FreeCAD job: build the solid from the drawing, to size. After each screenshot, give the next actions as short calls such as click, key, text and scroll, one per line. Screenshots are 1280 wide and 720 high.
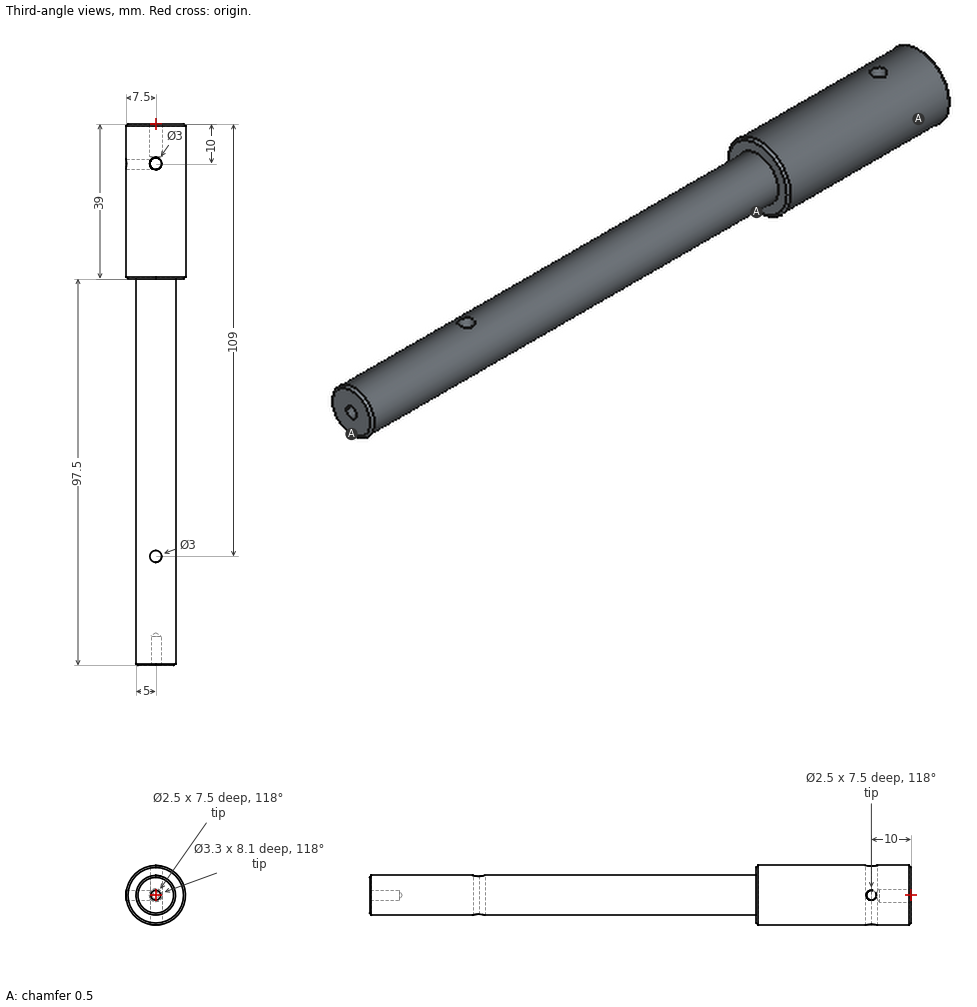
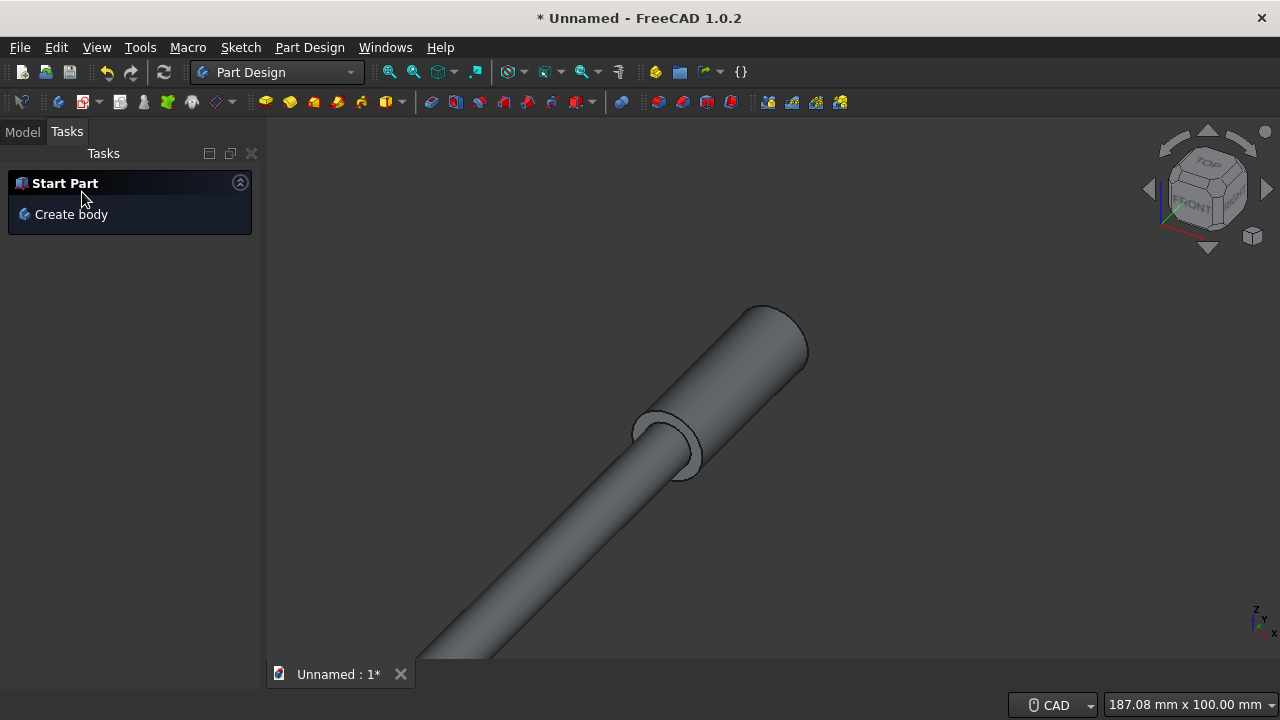
click(390, 72)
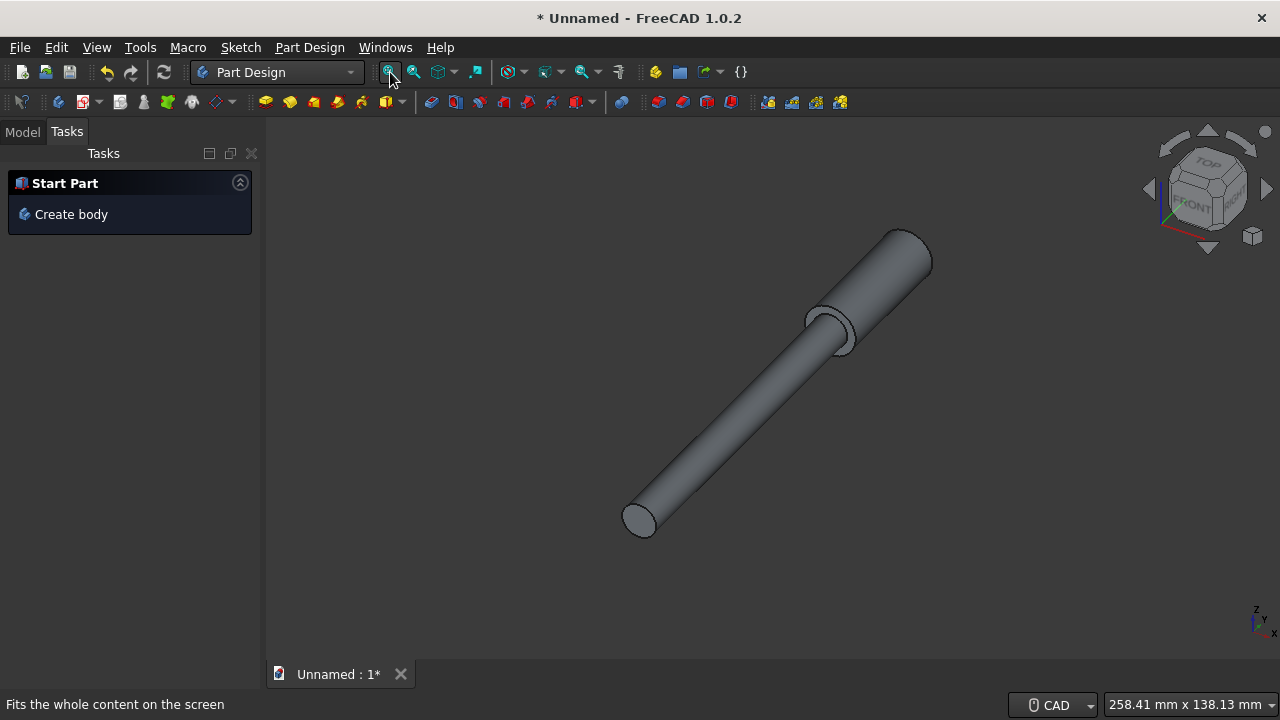
key(4)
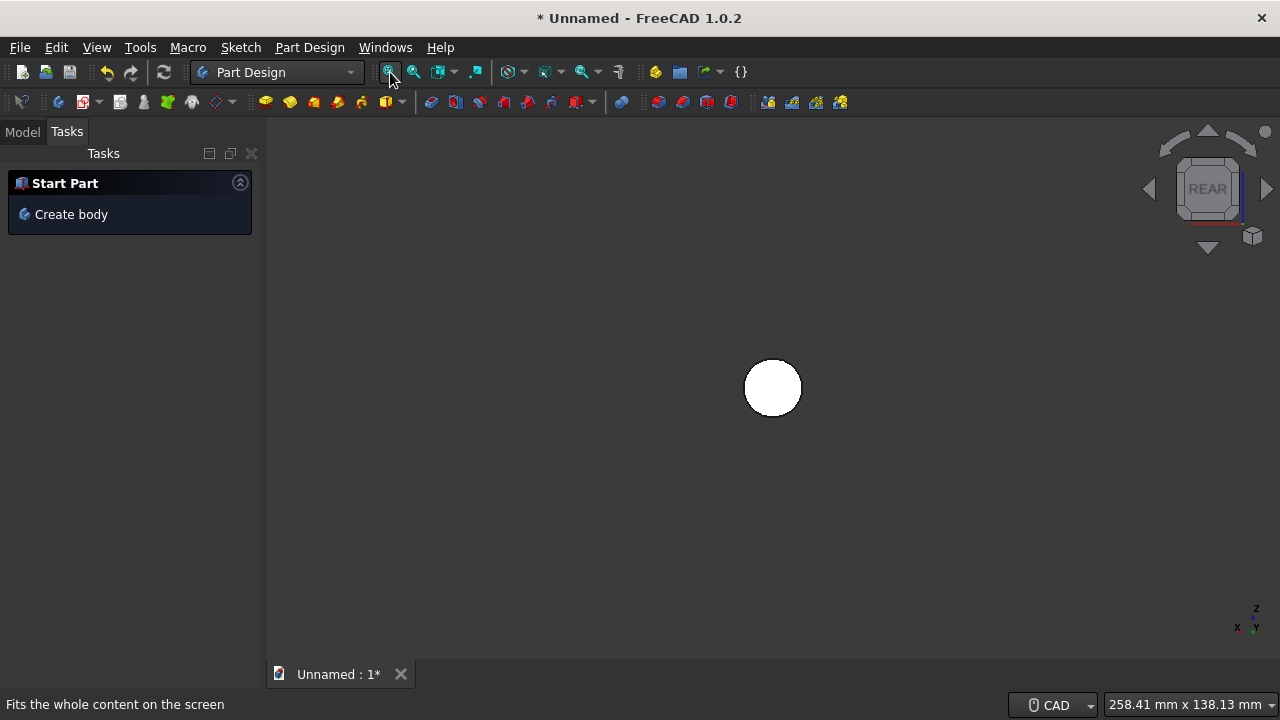
click(390, 72)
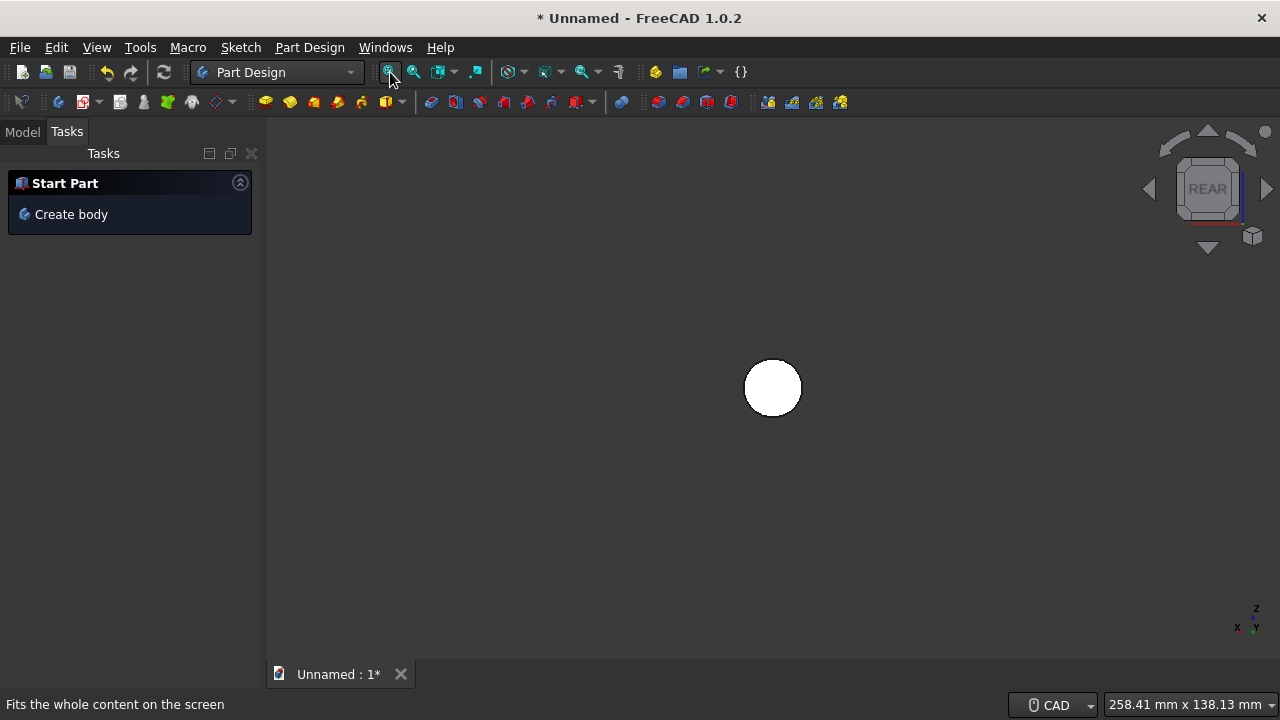
click(773, 387)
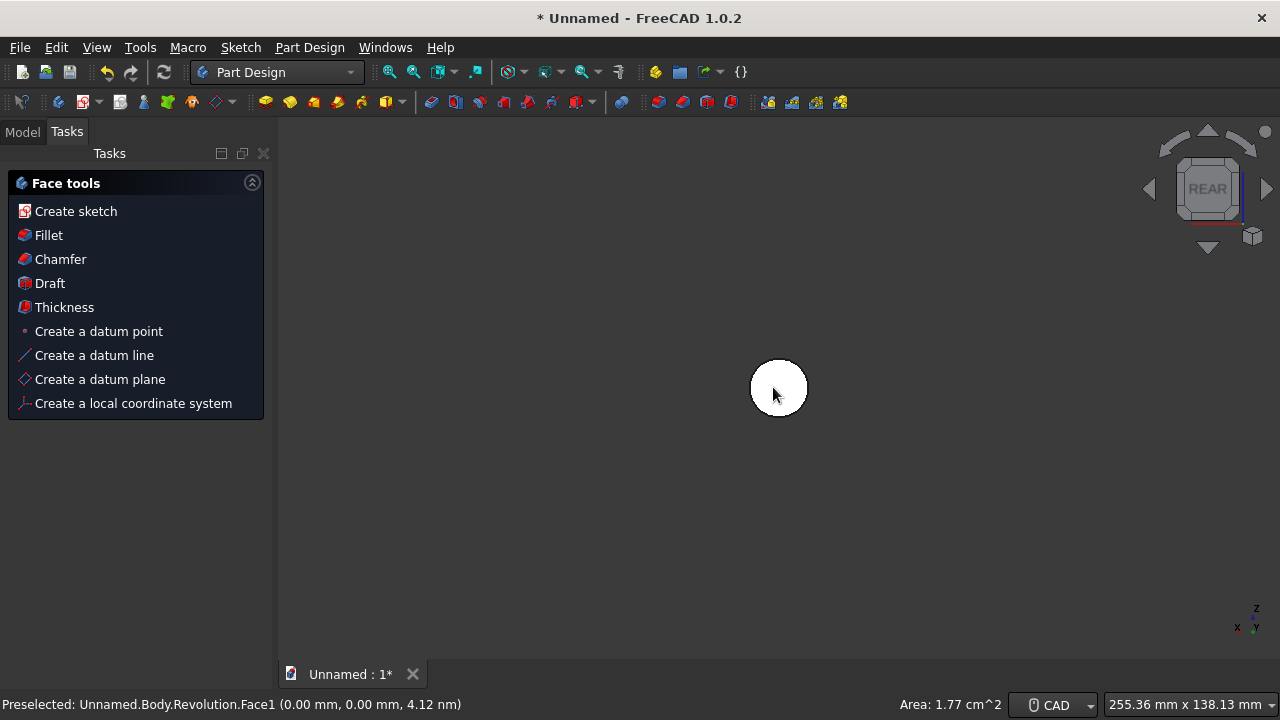
click(84, 102)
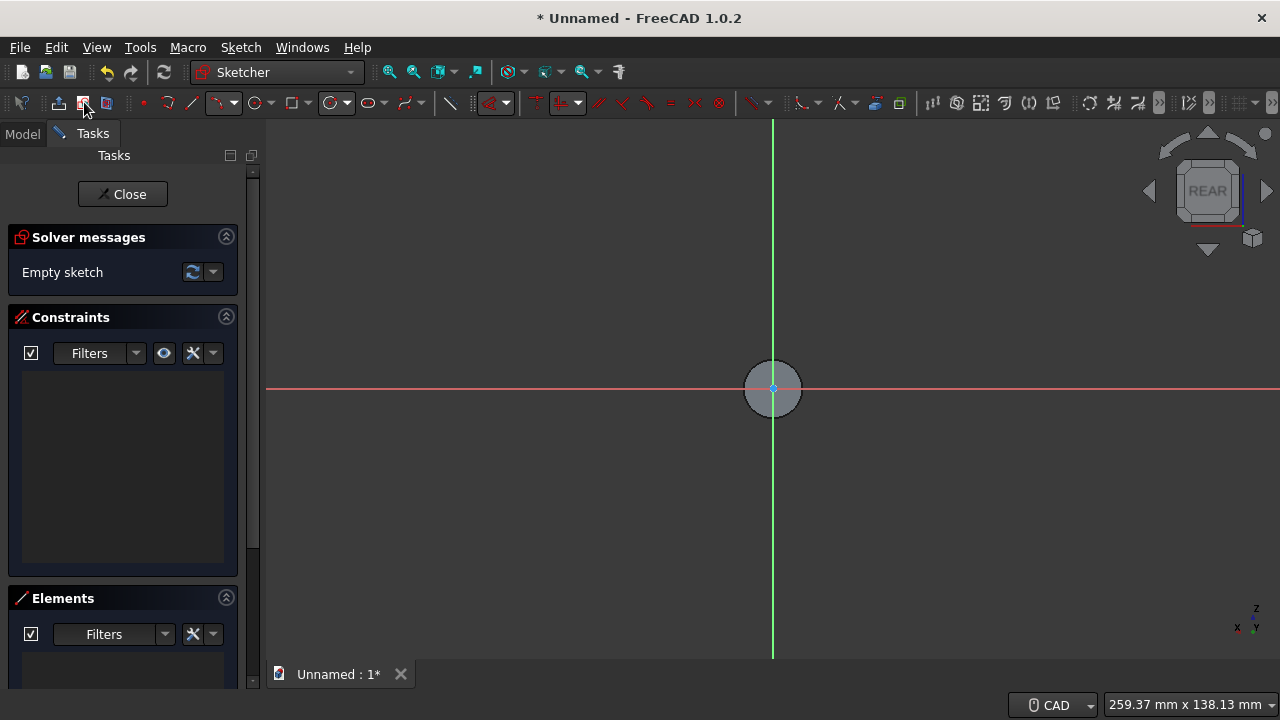
scroll(777, 389, up, 15)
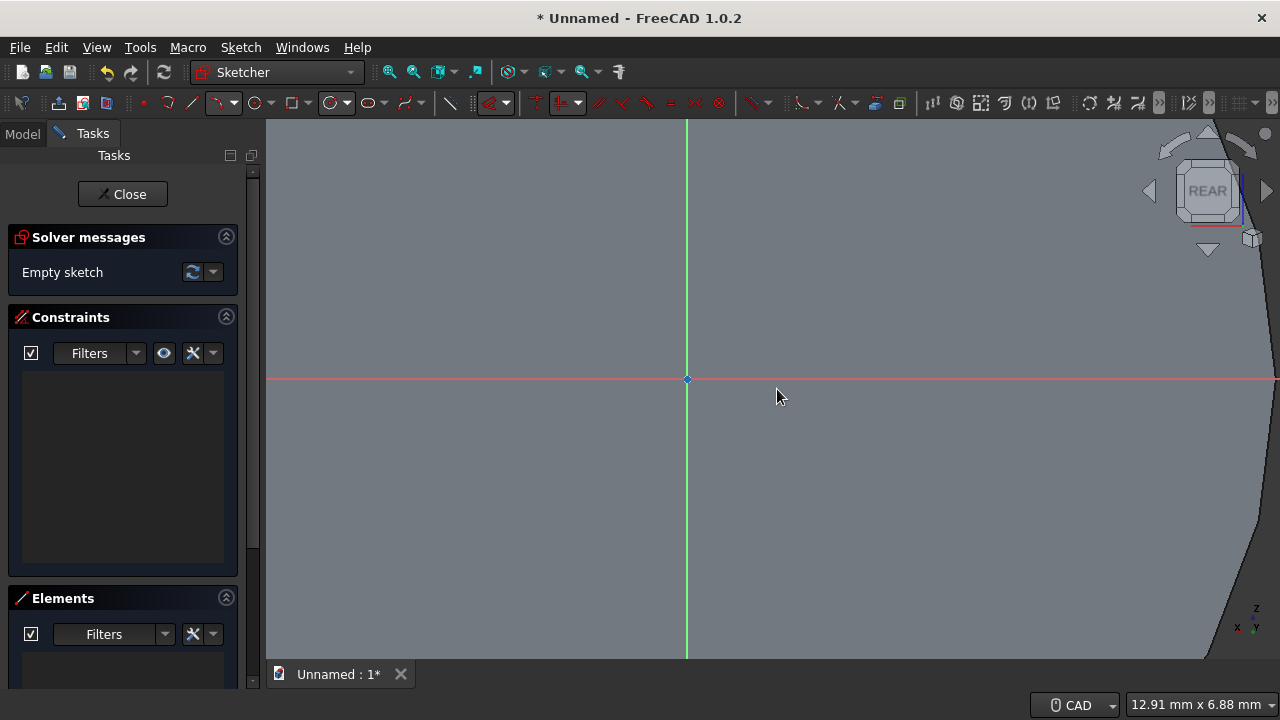
click(256, 104)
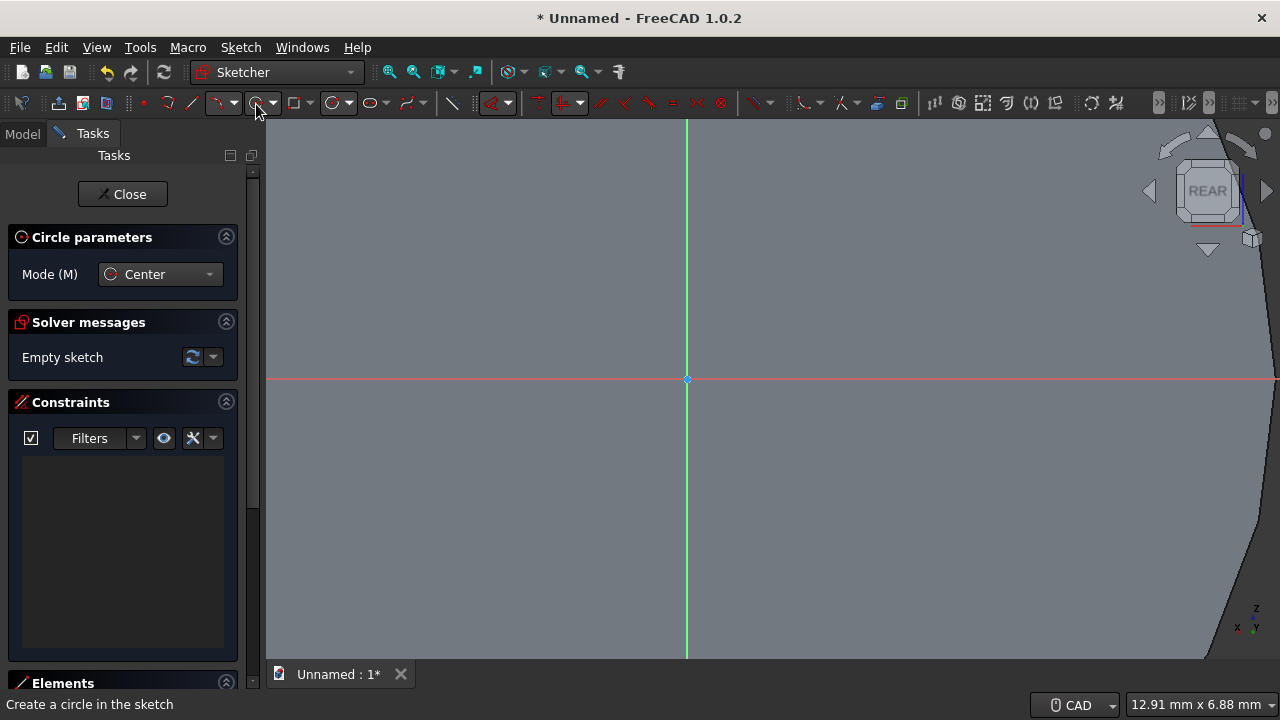
click(687, 379)
click(779, 288)
key(Escape)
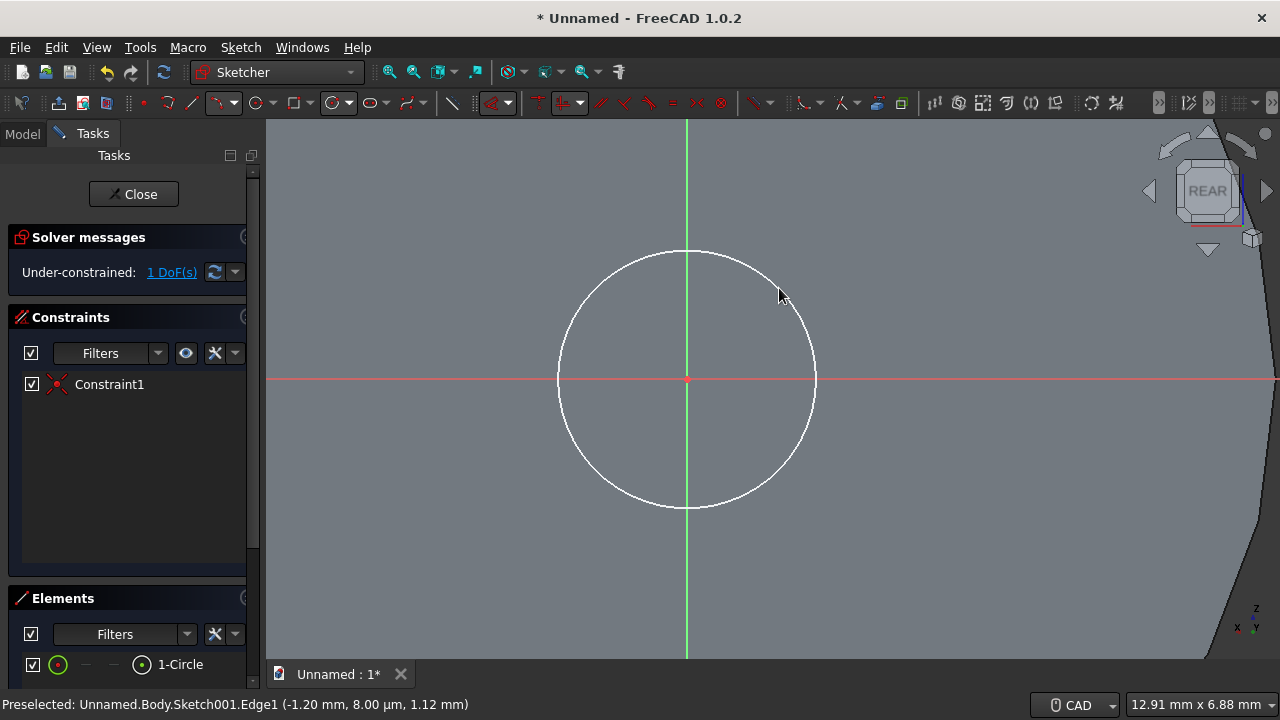
click(778, 288)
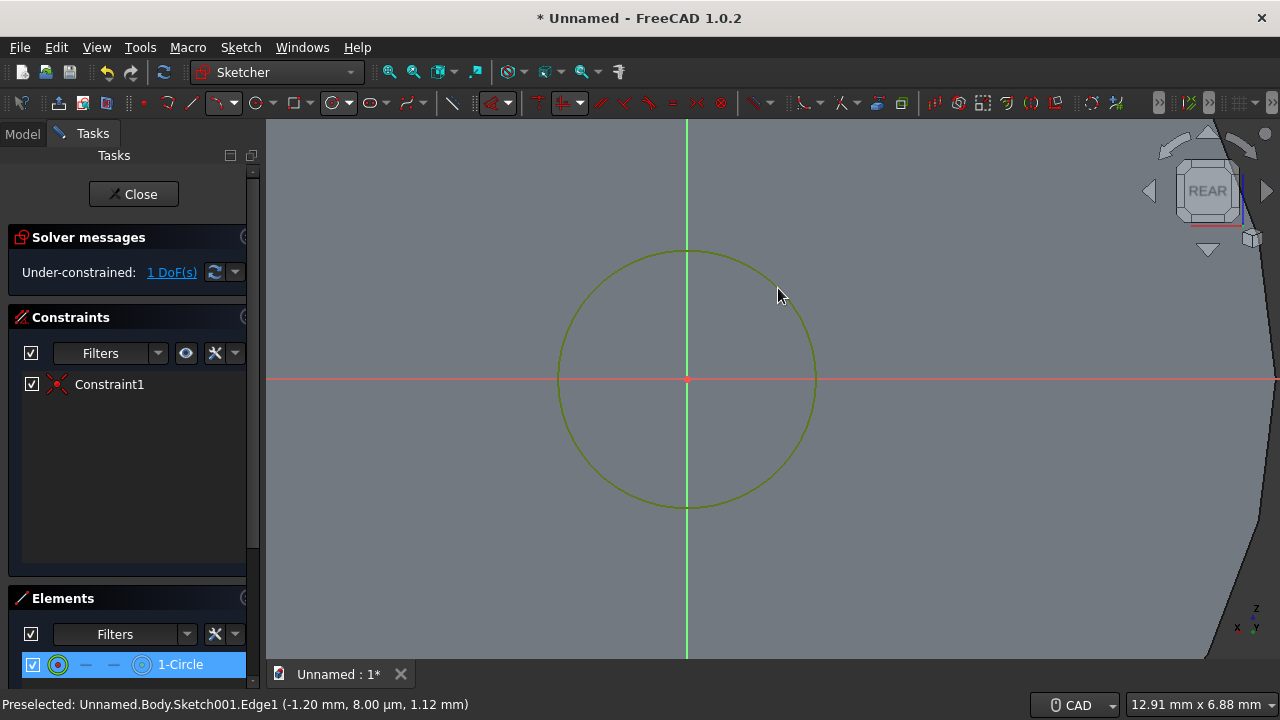
key(k)
key(o)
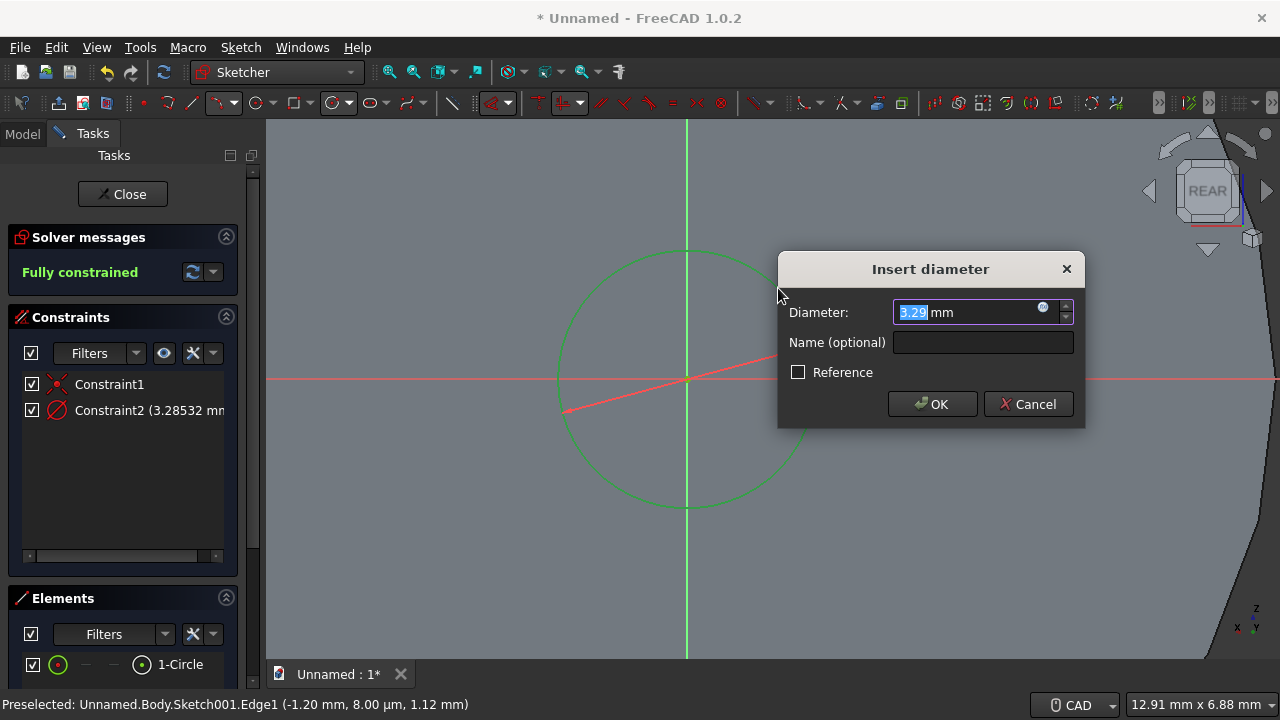
text(3.3)
key(Return)